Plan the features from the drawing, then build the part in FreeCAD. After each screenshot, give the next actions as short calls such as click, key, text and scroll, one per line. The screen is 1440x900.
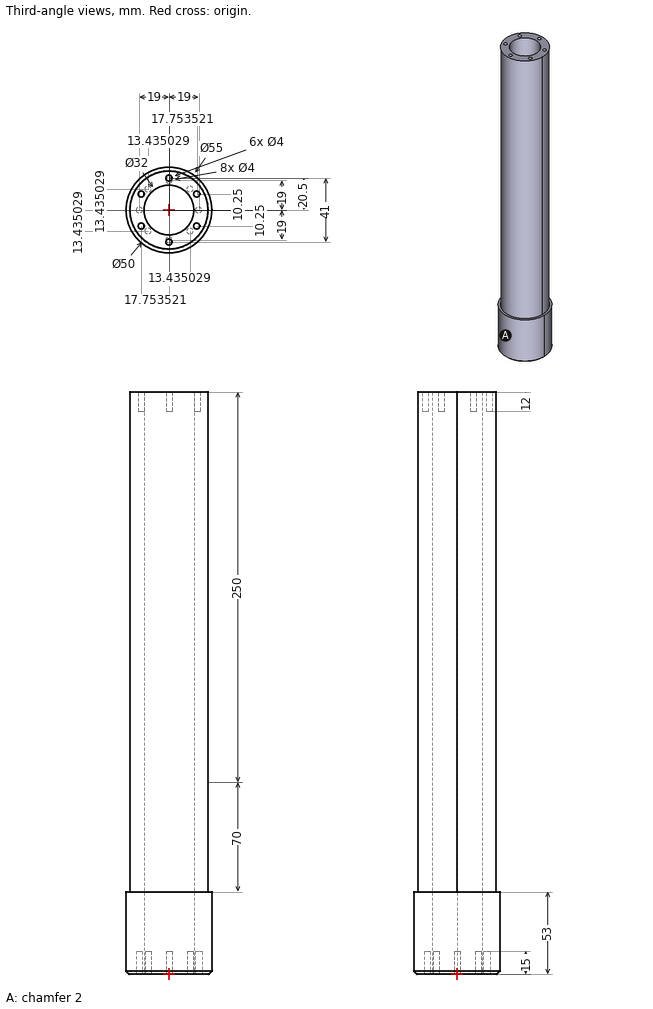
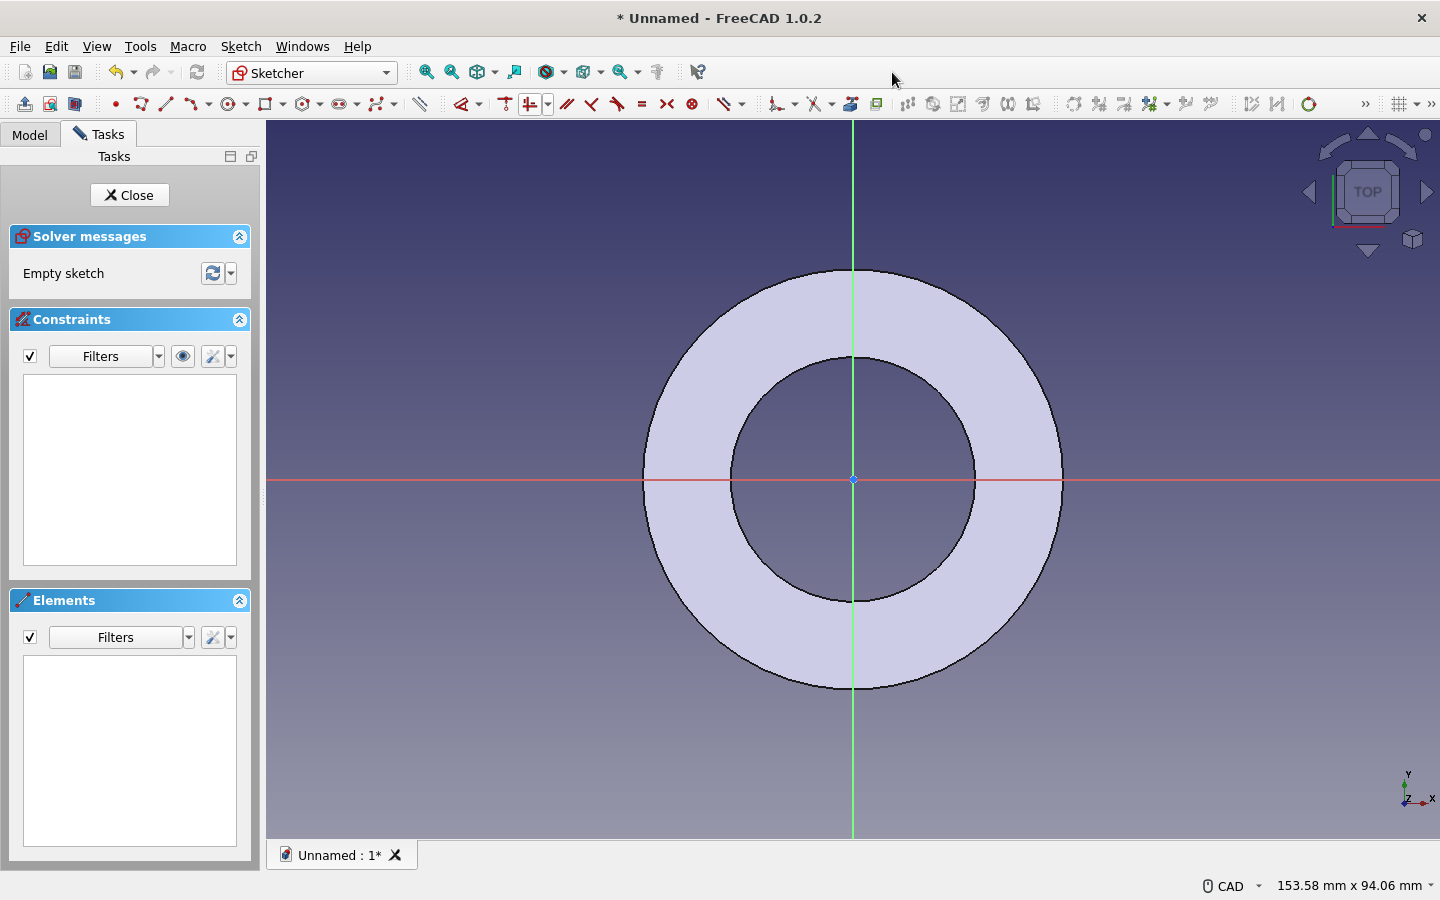
click(228, 104)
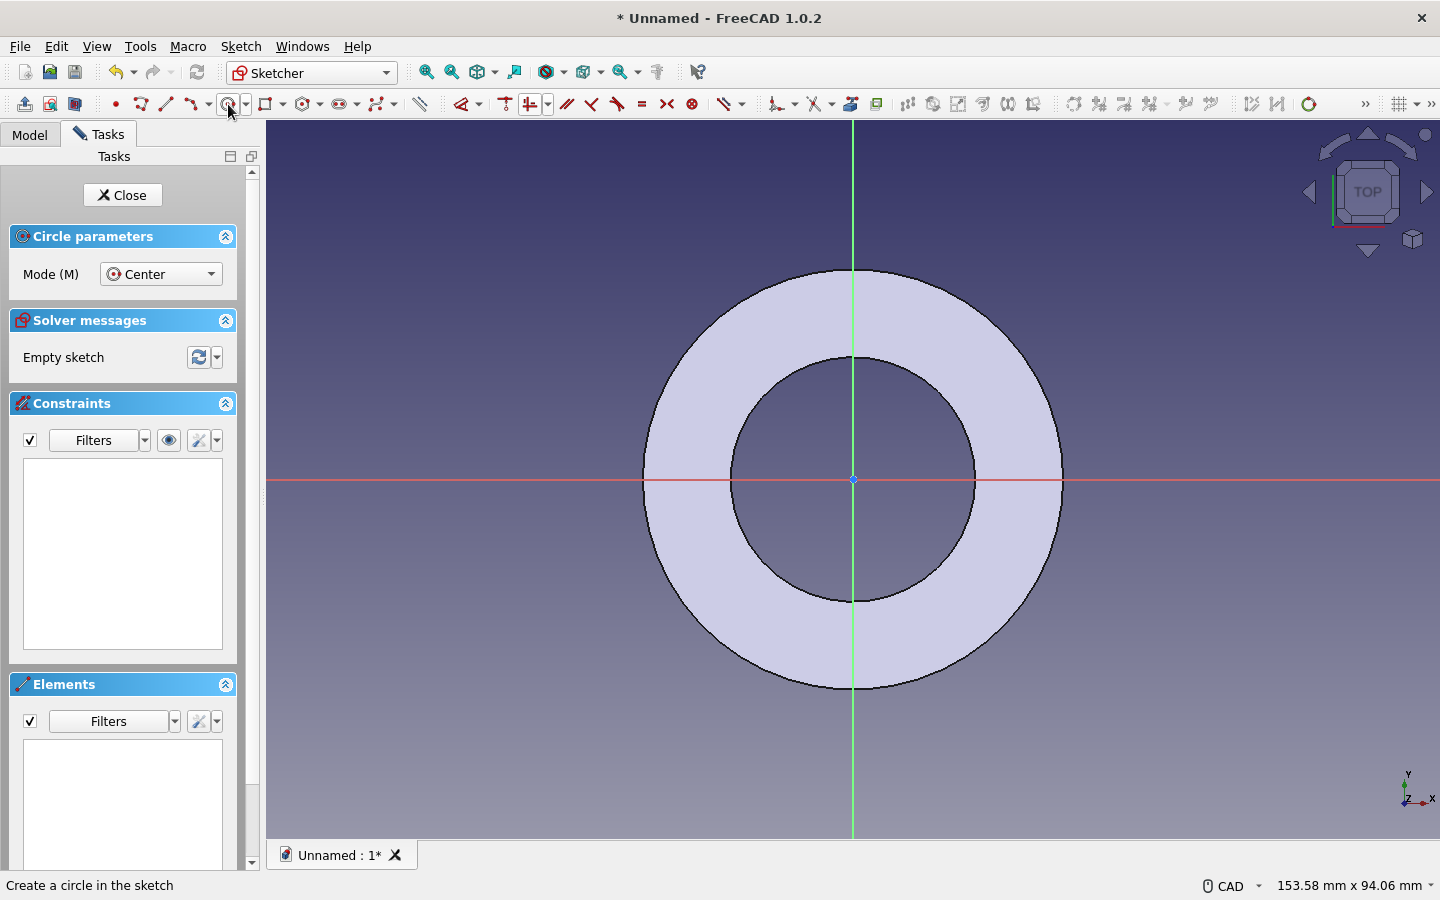
click(853, 480)
move(988, 344)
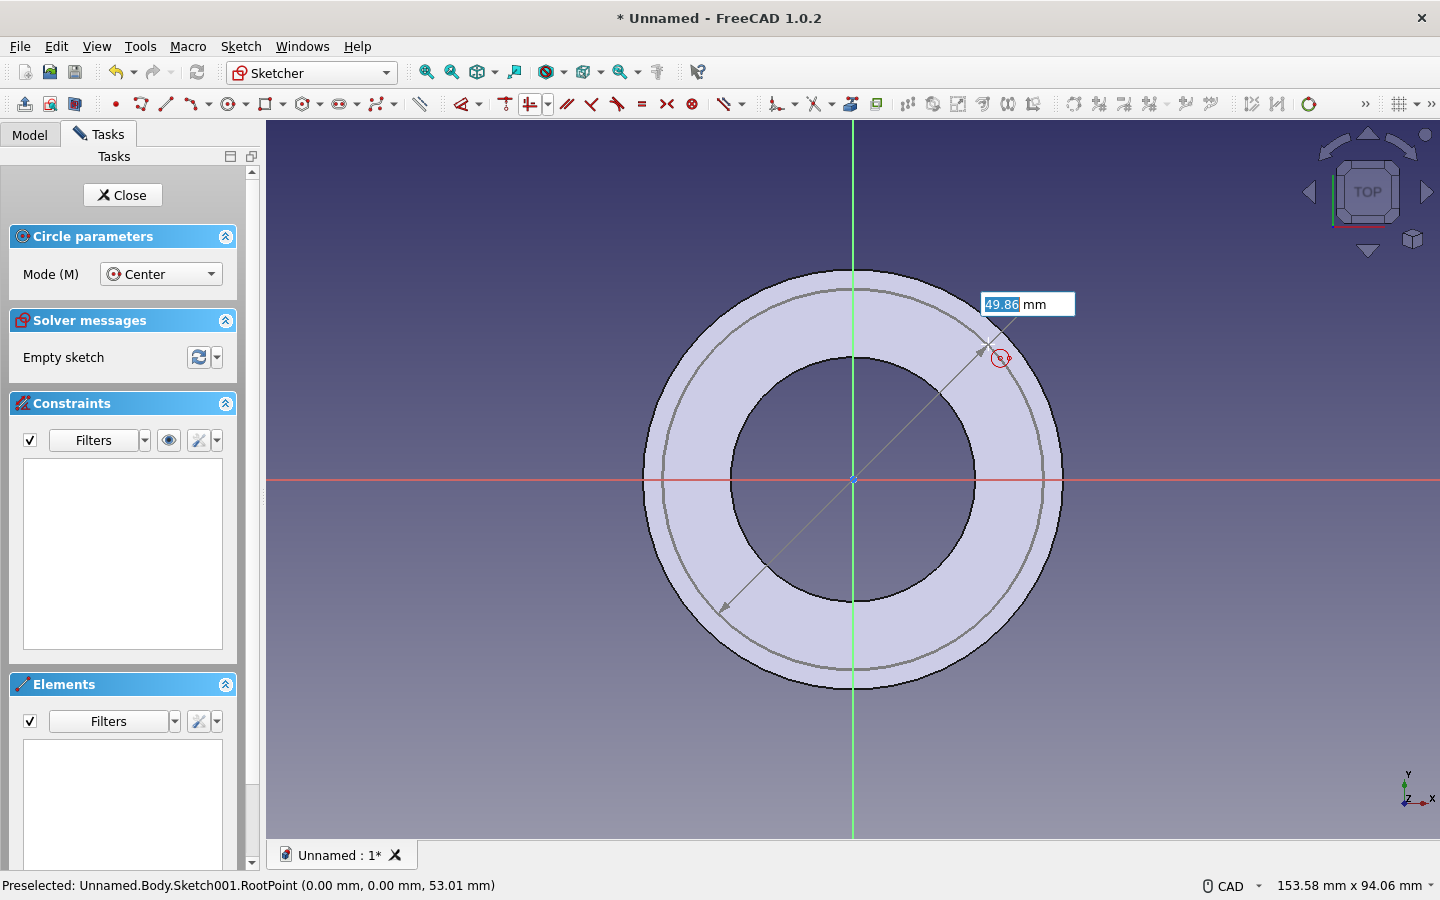
text(50)
key(Return)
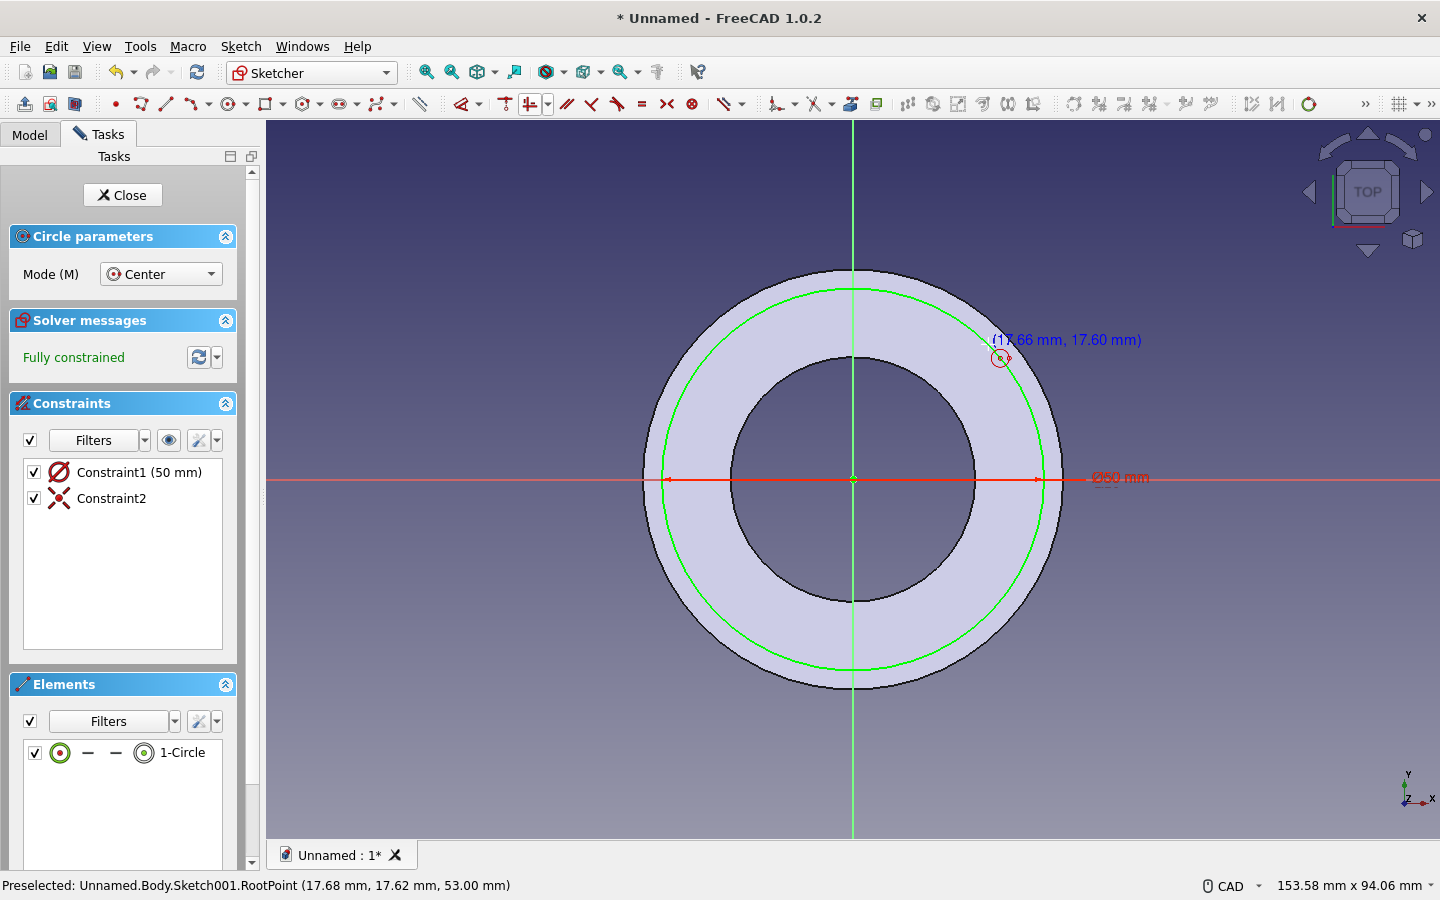
click(853, 480)
move(939, 393)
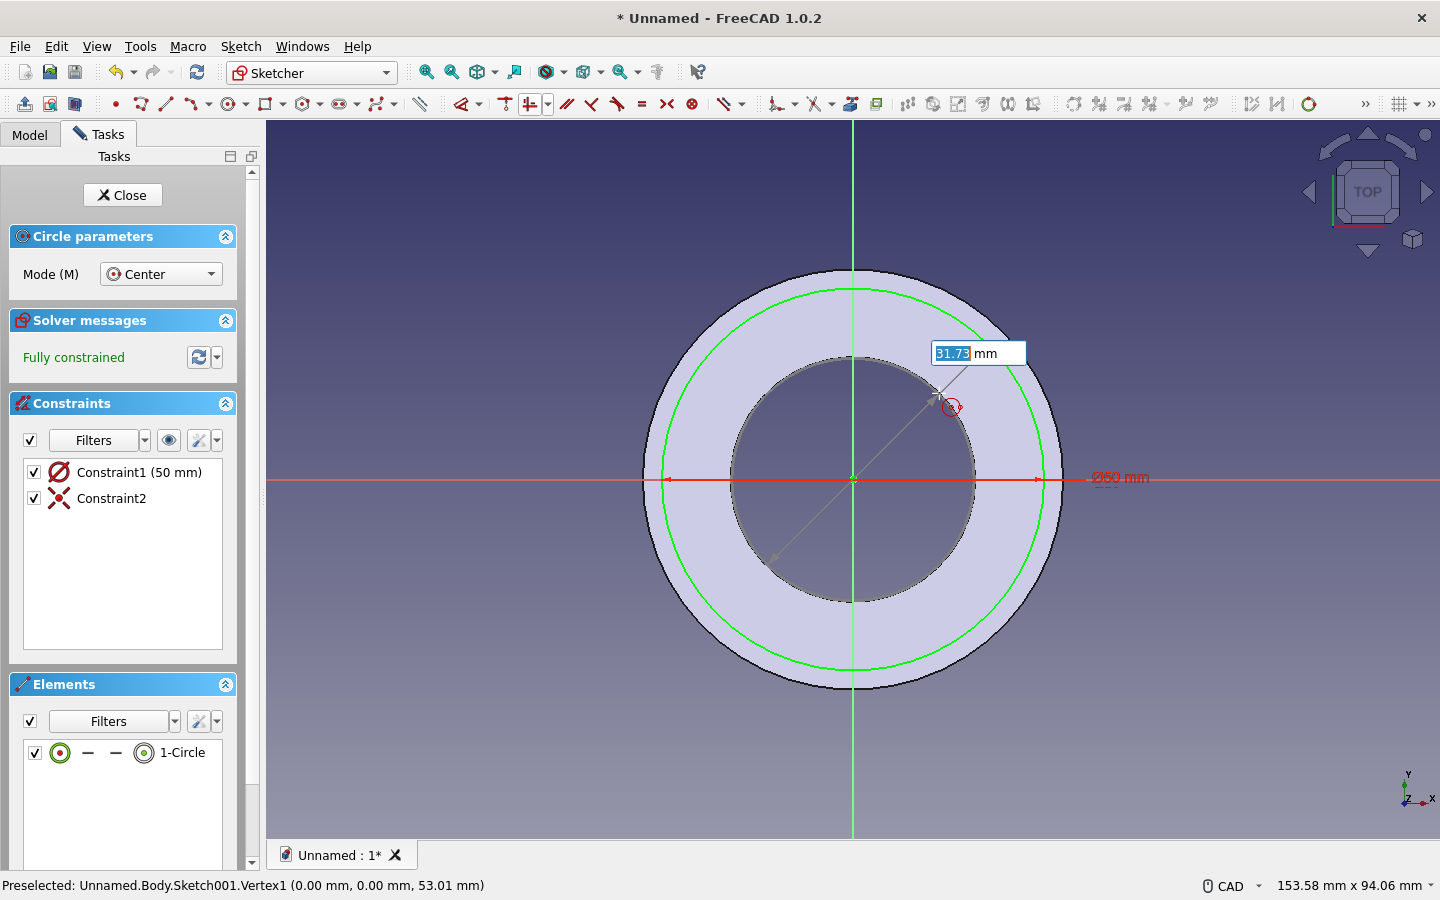
text(32)
key(Return)
key(Escape)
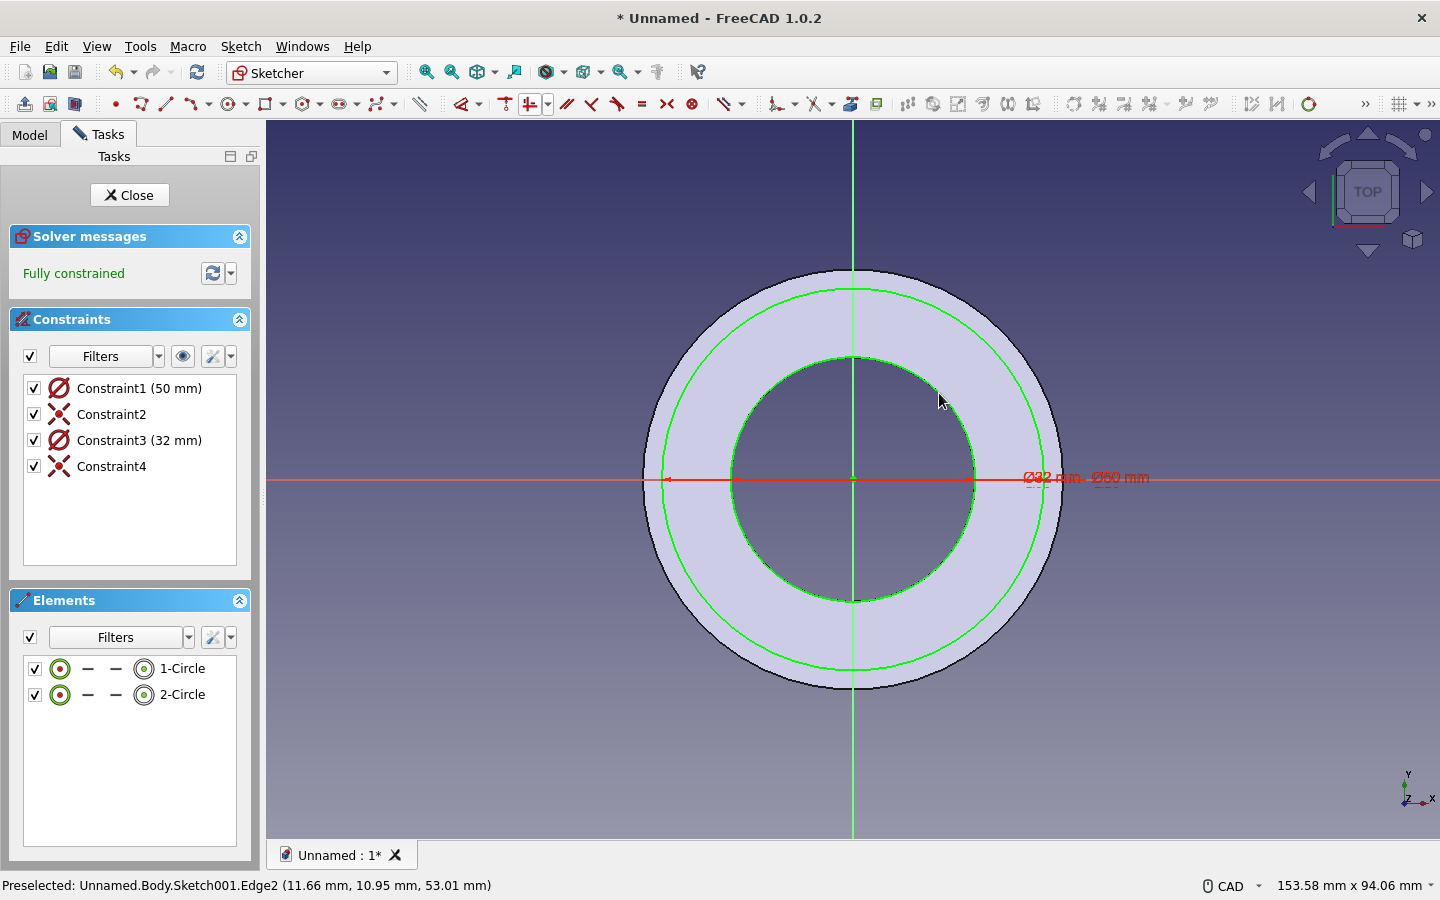
click(130, 195)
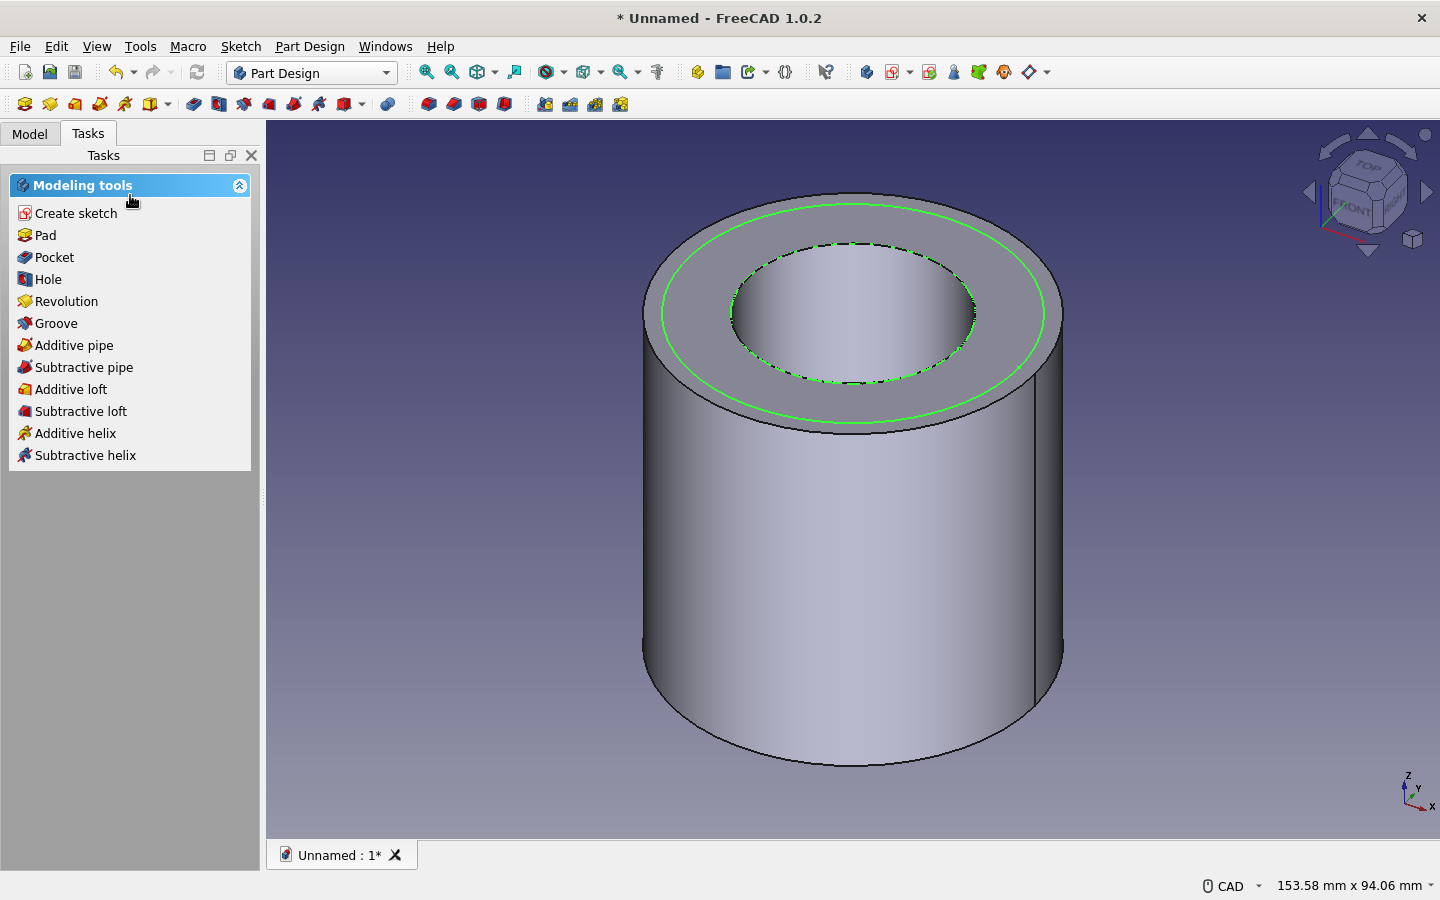
click(25, 104)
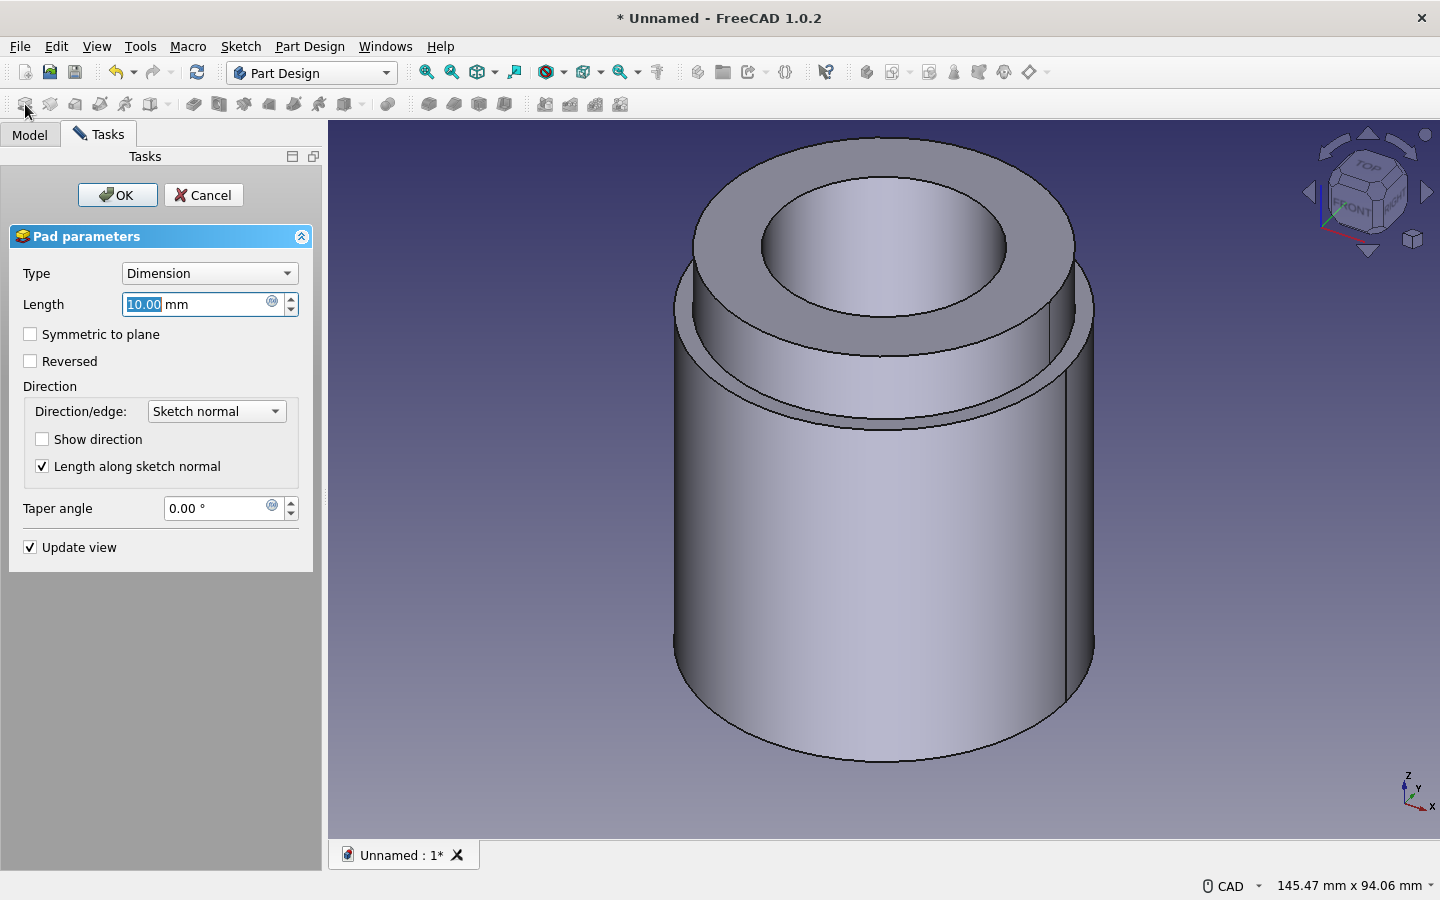
text(70)
key(Tab)